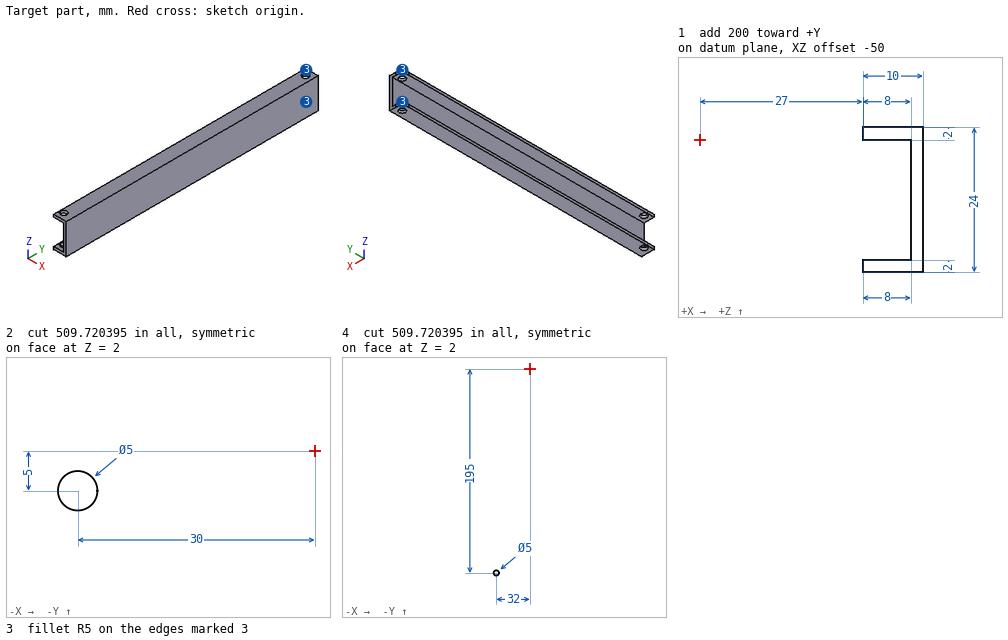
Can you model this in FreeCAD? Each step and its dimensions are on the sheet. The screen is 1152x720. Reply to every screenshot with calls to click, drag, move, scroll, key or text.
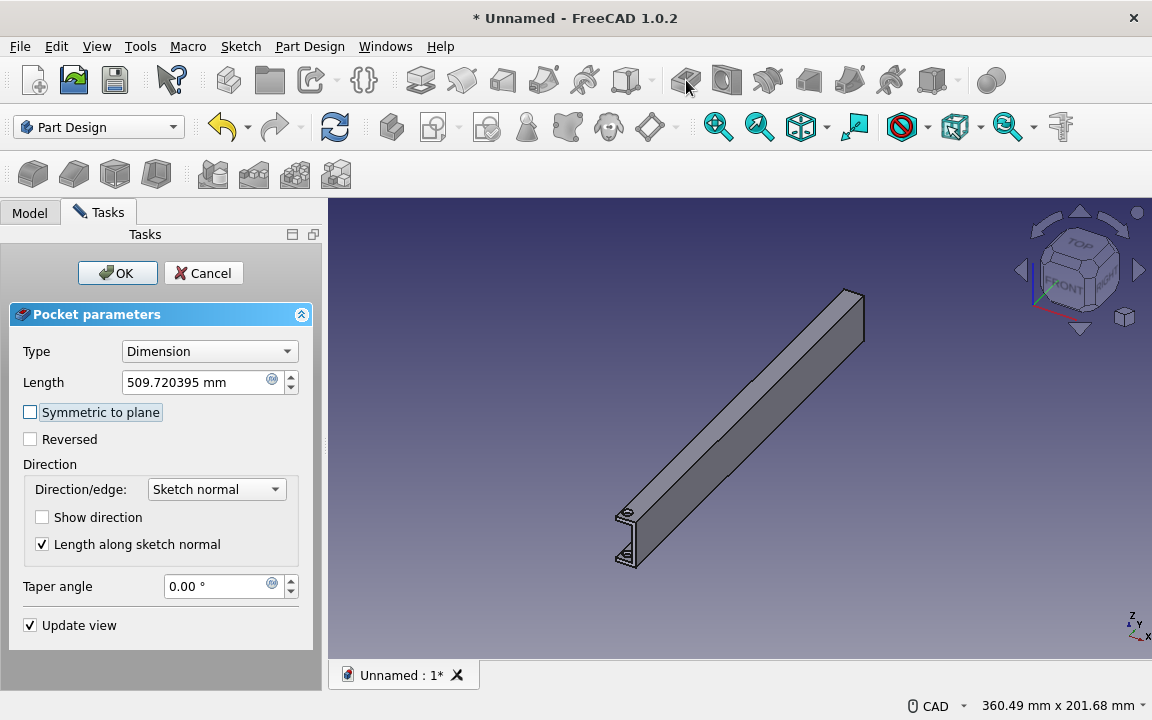
click(31, 412)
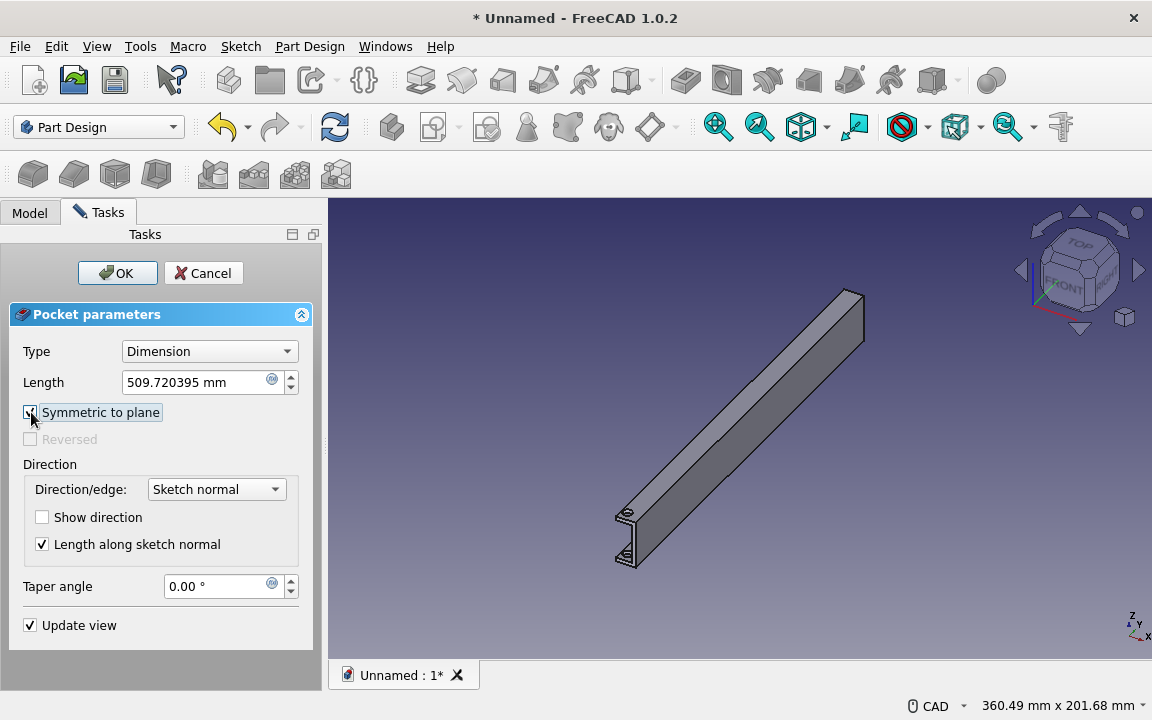
click(118, 273)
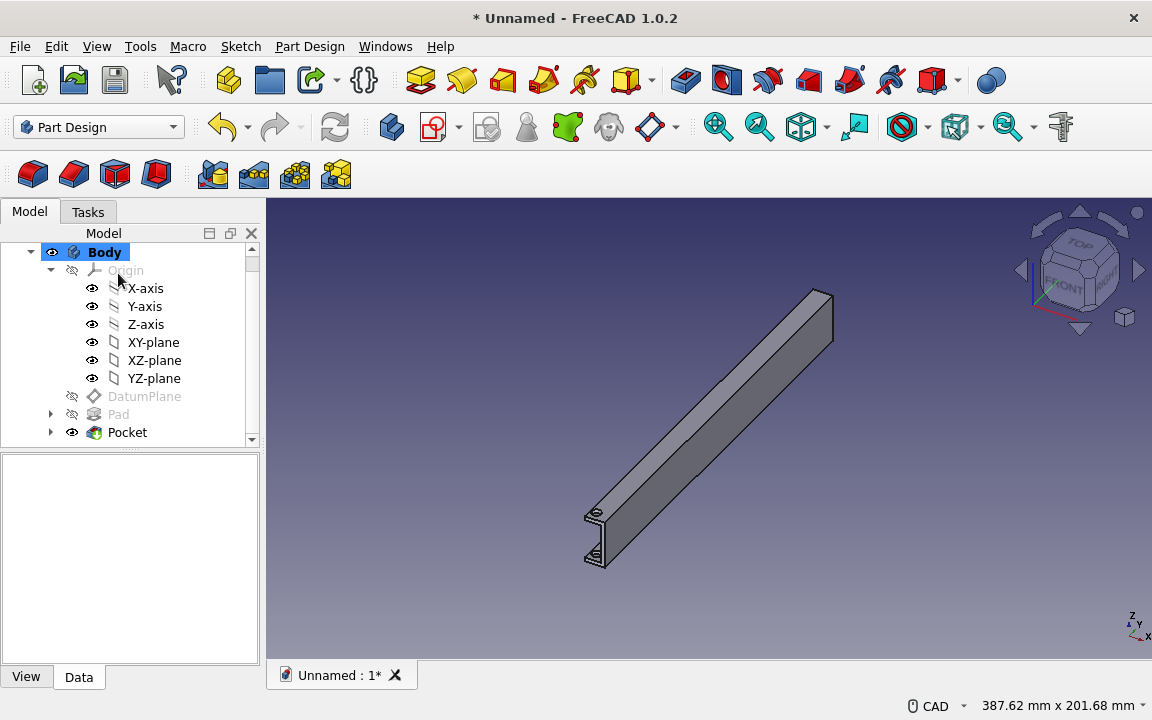
scroll(813, 290, up, 11)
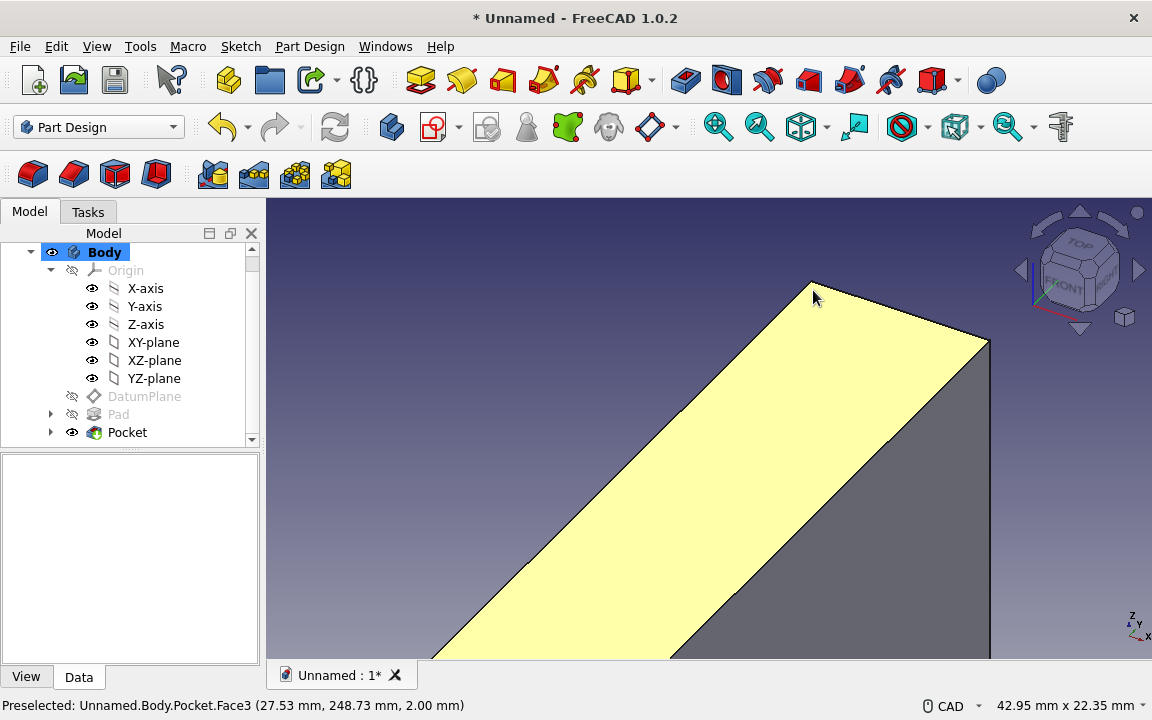
click(719, 128)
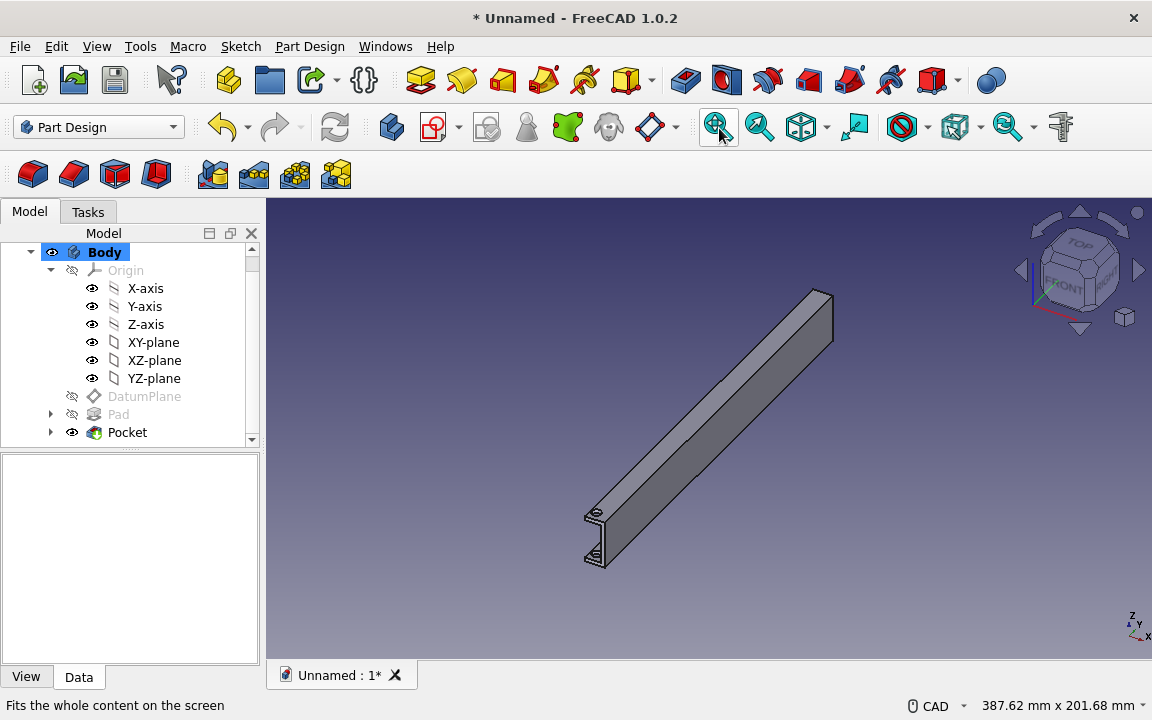
key(0)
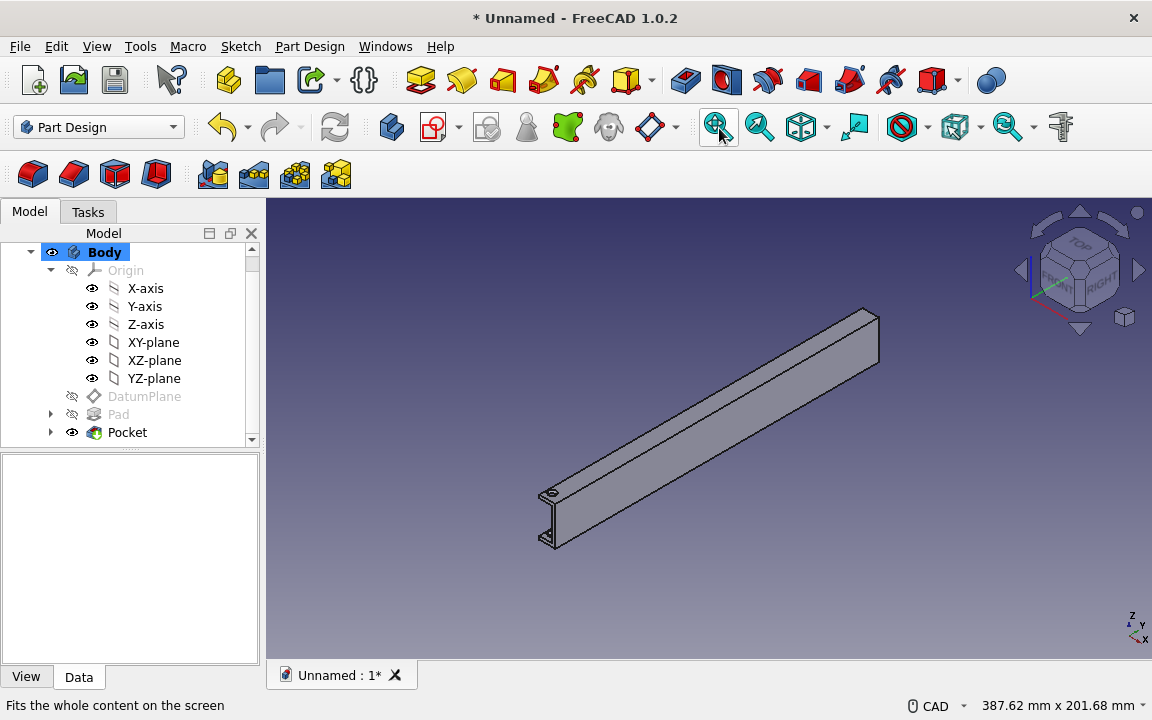
scroll(863, 309, up, 11)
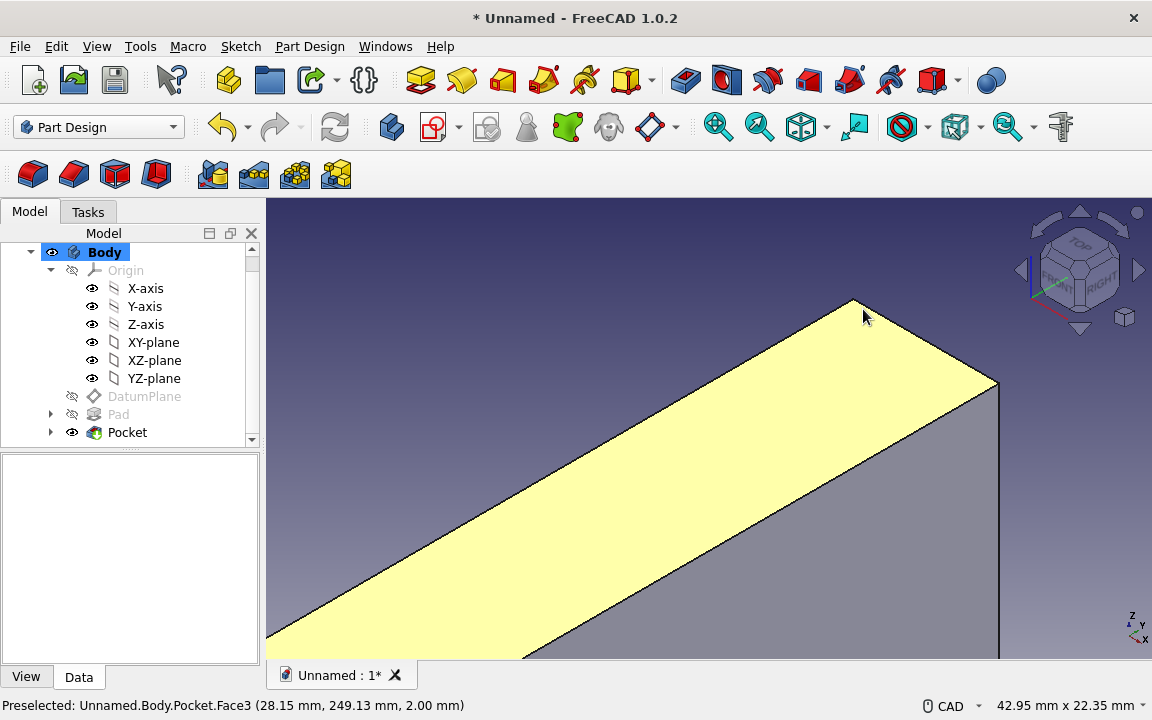
click(719, 128)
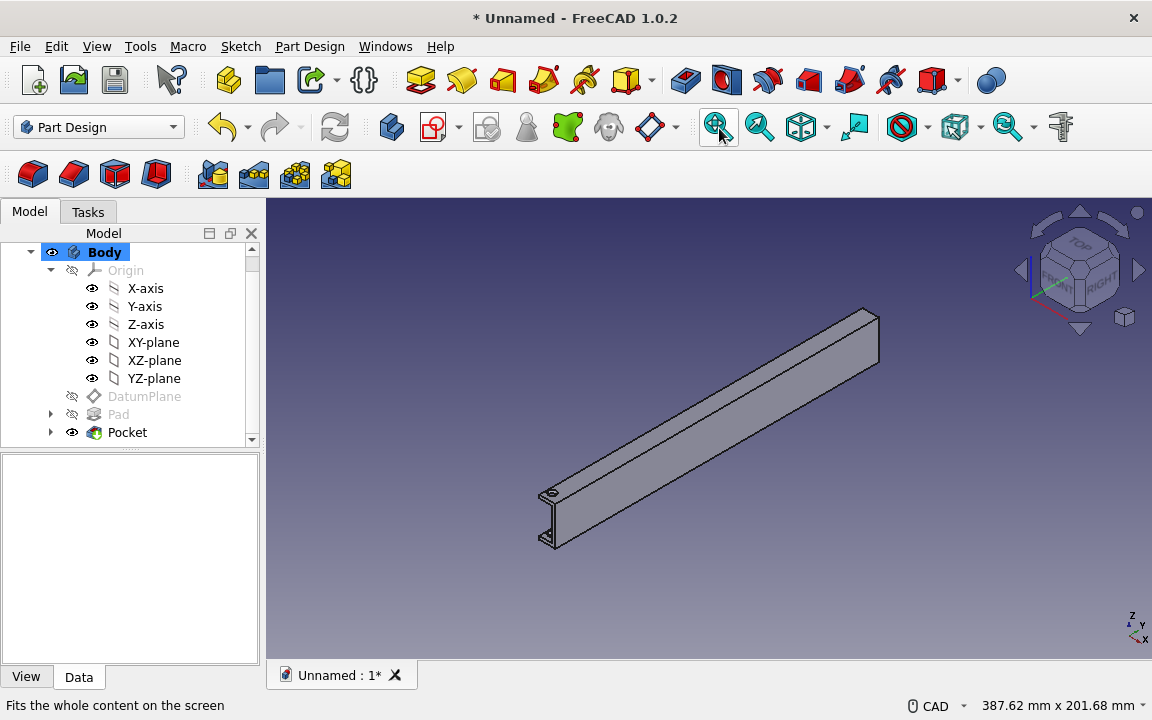
key(2)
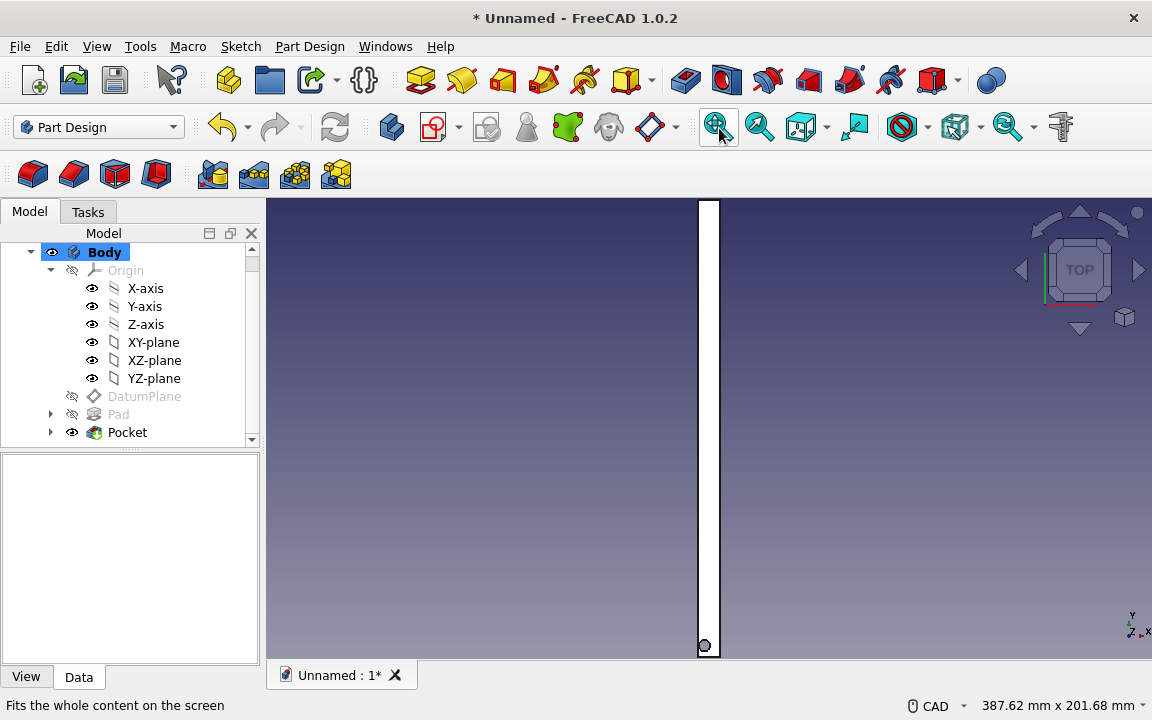
key(1)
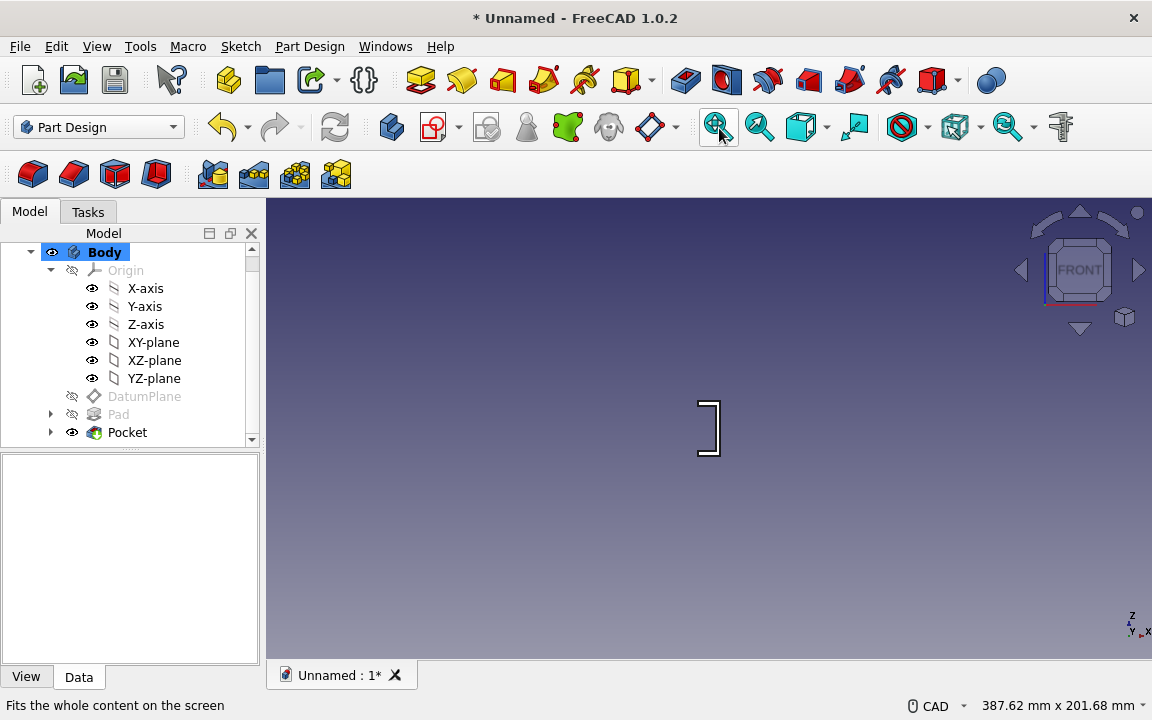
click(719, 128)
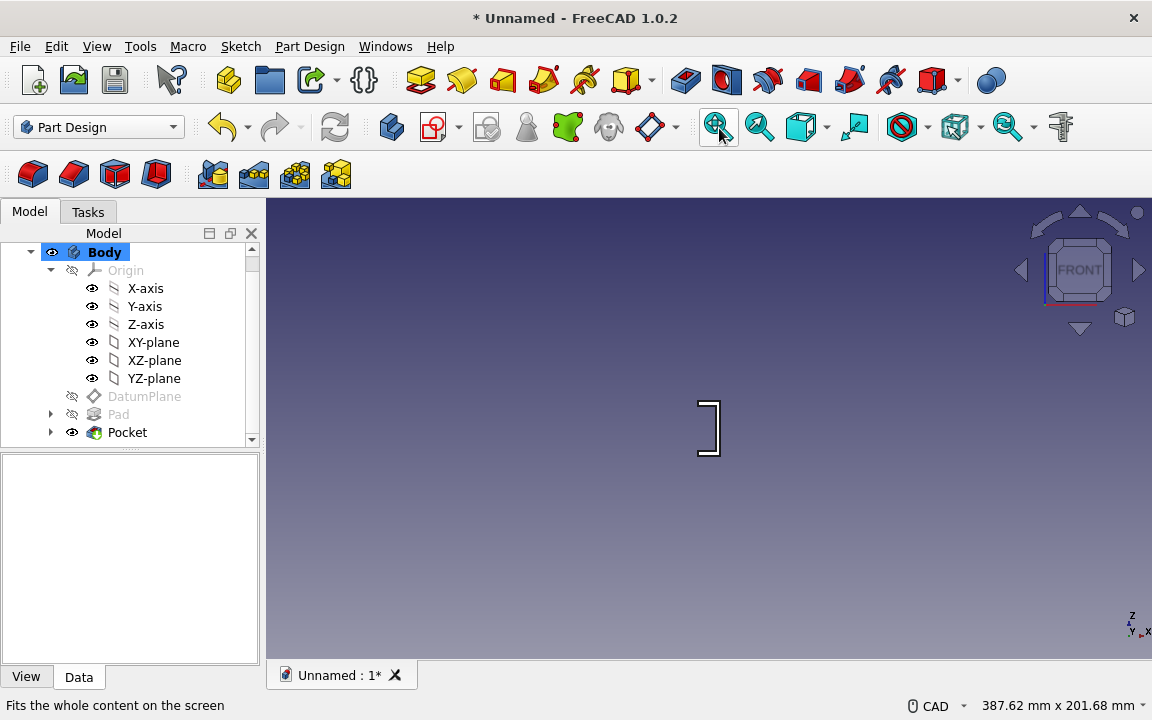
scroll(698, 402, up, 11)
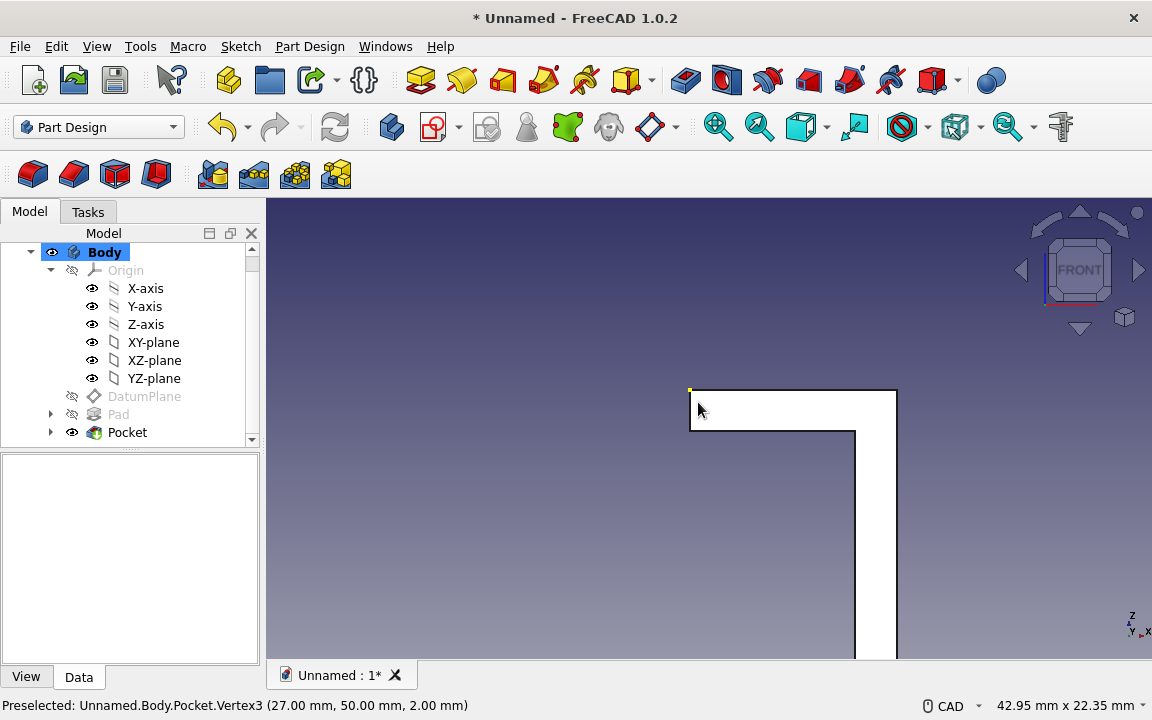
click(719, 128)